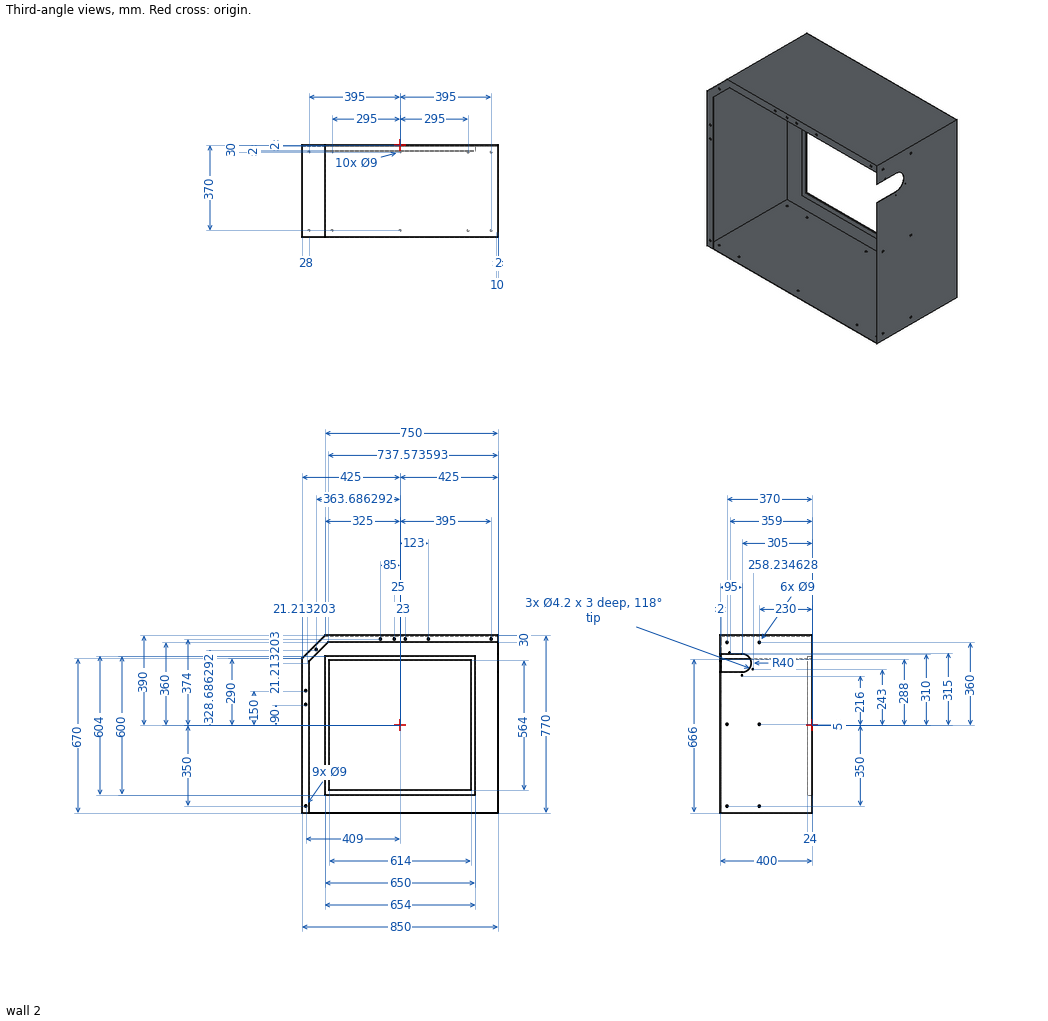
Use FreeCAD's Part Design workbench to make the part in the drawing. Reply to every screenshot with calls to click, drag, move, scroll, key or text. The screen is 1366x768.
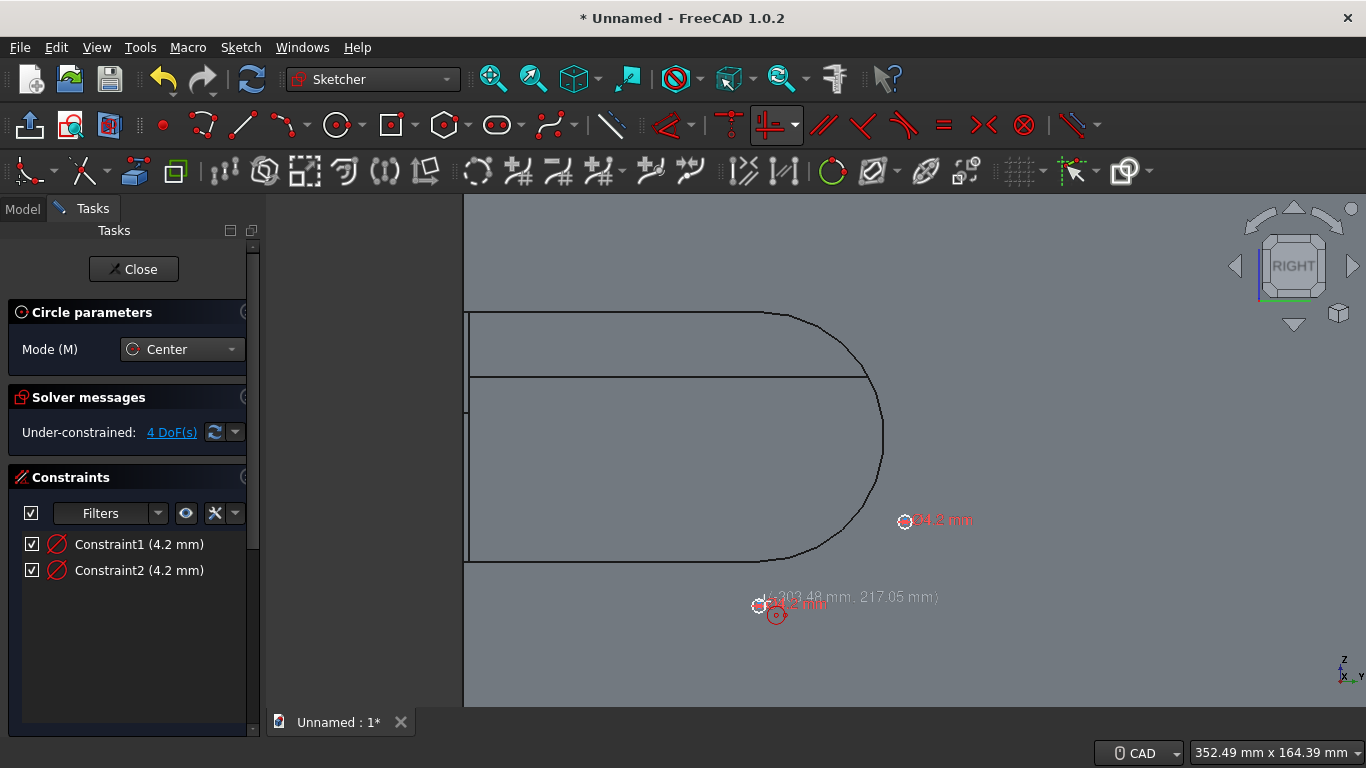
scroll(591, 296, up, 7)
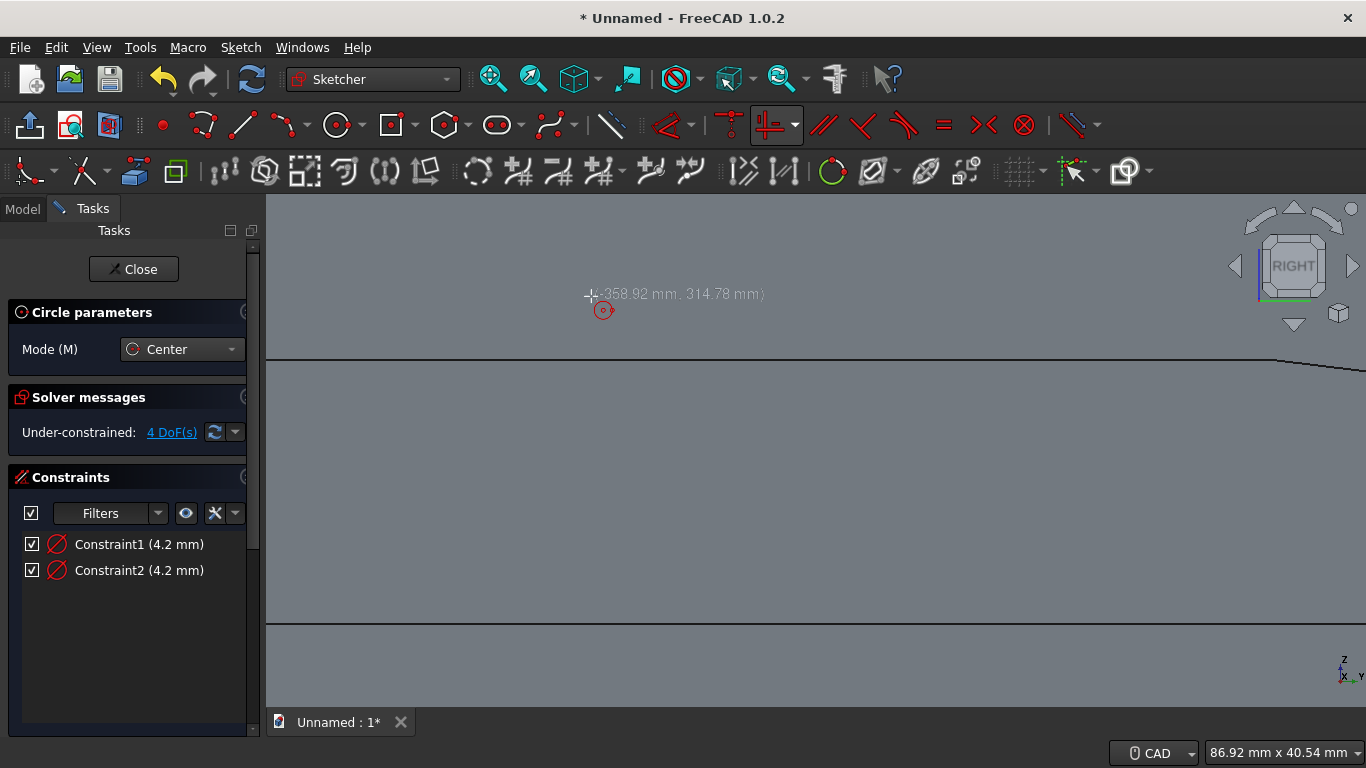
scroll(591, 296, down, 7)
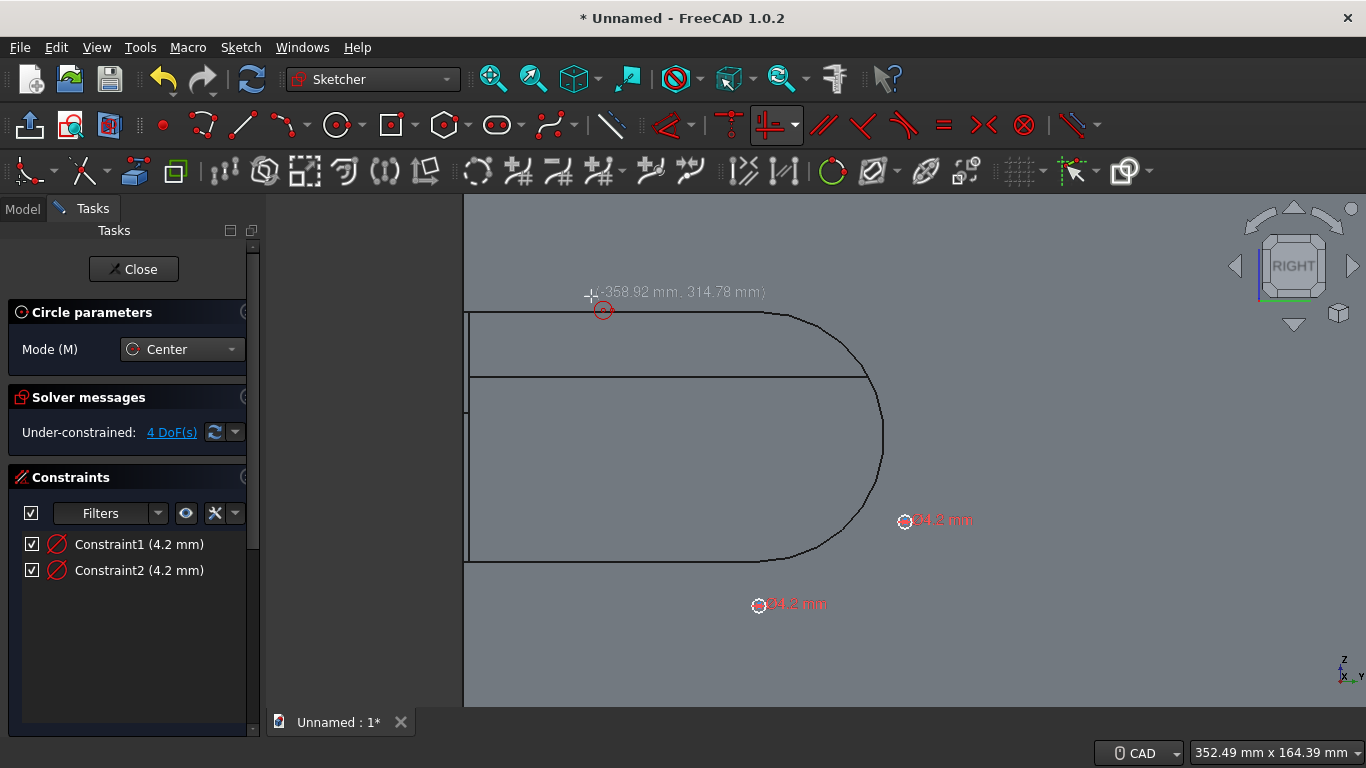
click(591, 296)
move(595, 292)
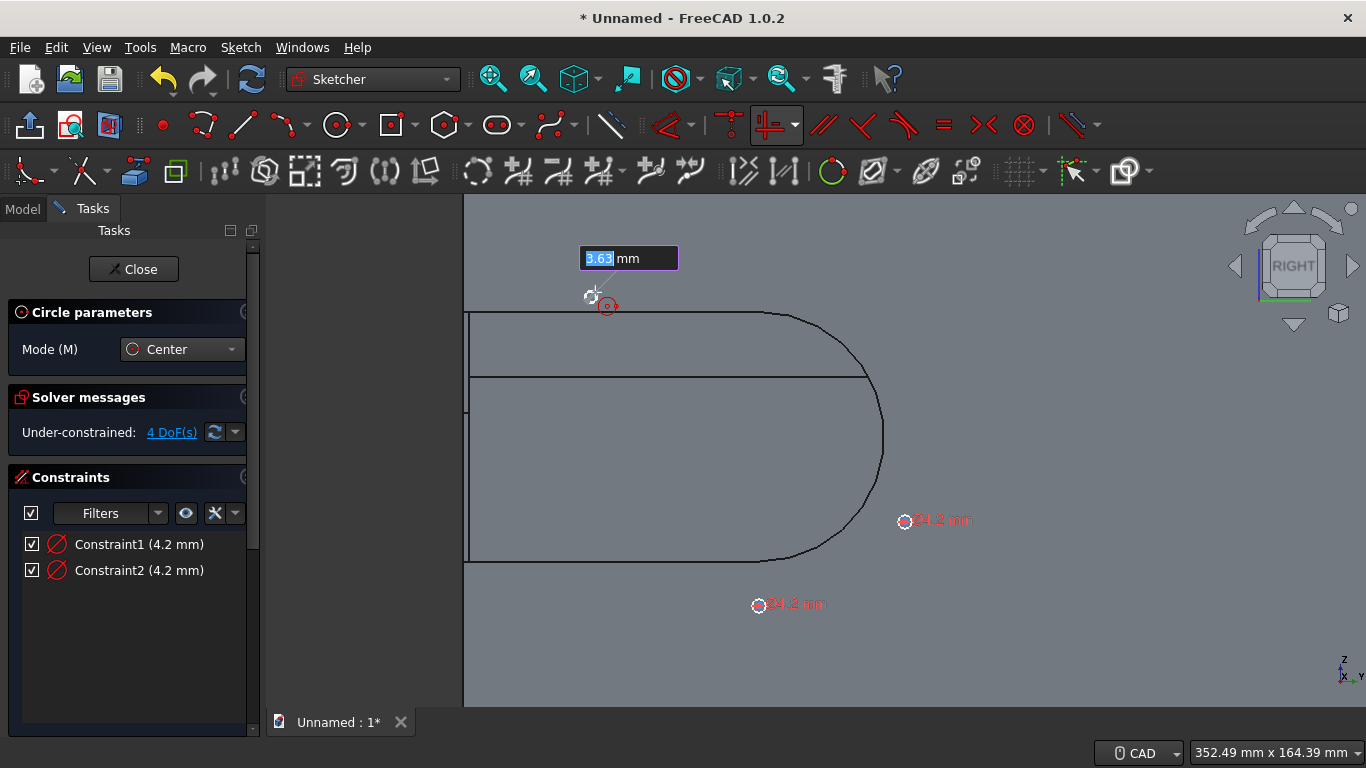
text(4.2)
key(Return)
key(Escape)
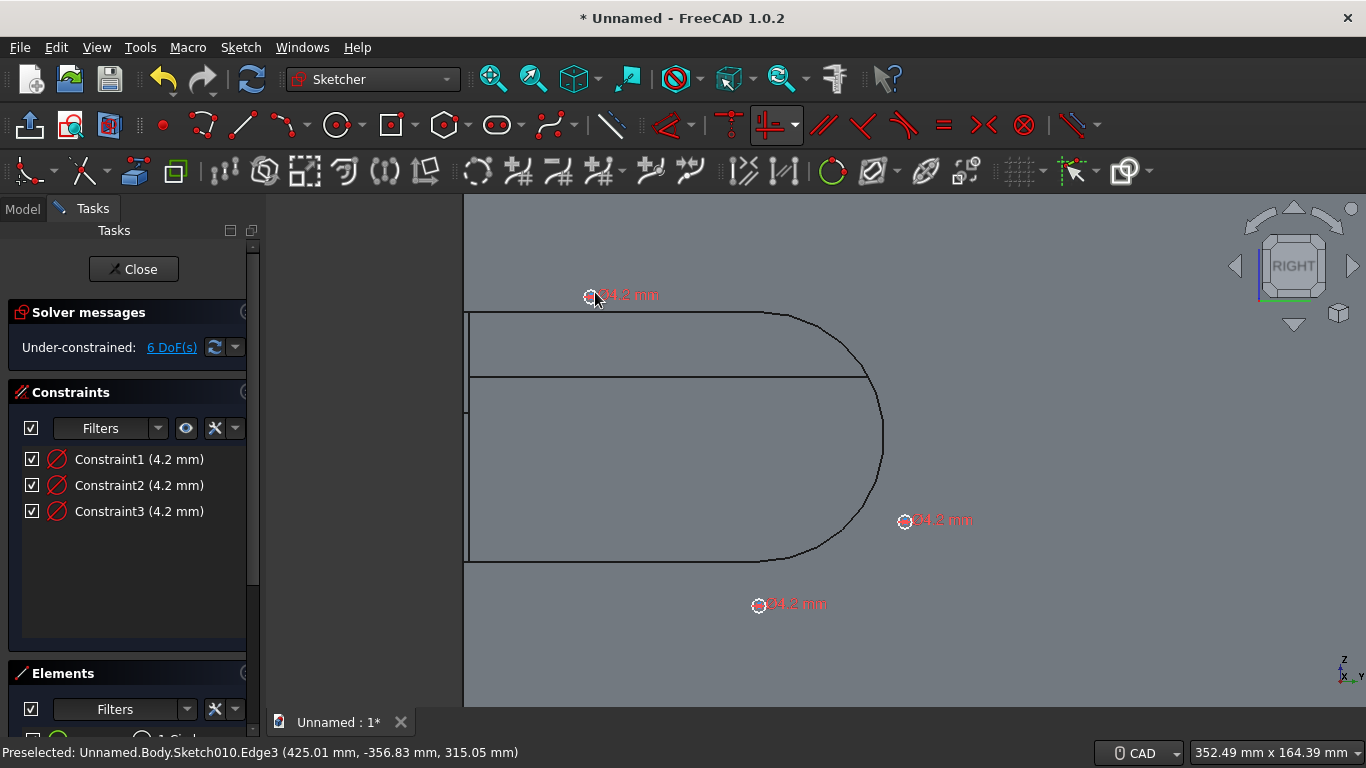
click(666, 126)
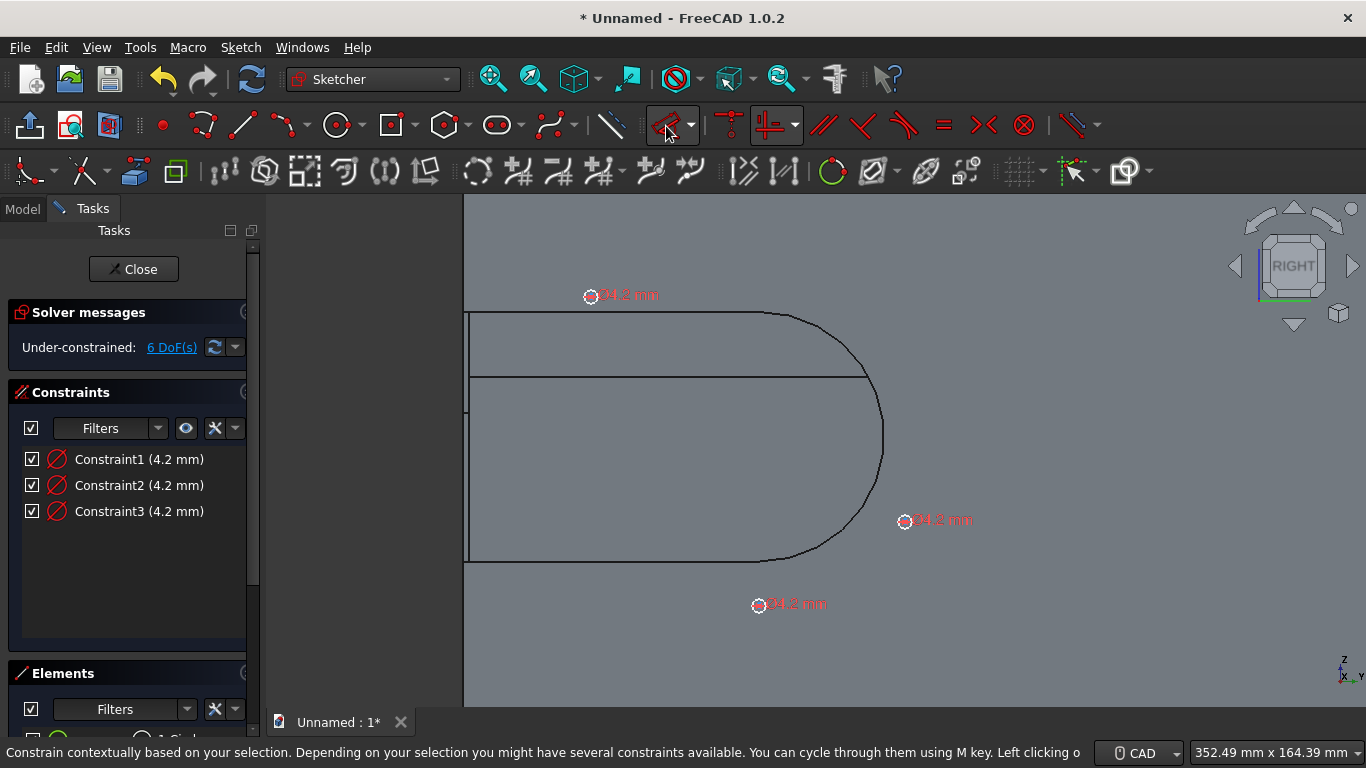
click(905, 522)
click(871, 600)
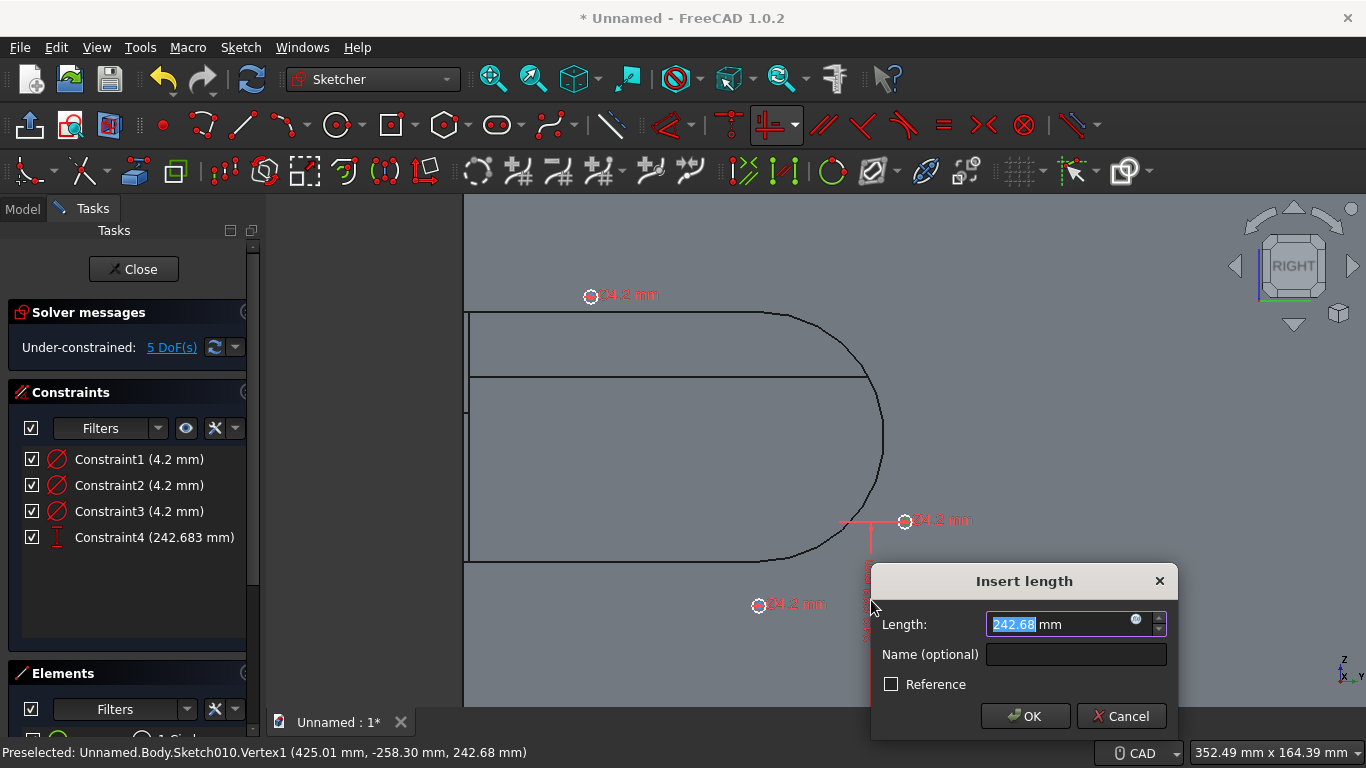
text(243)
key(Return)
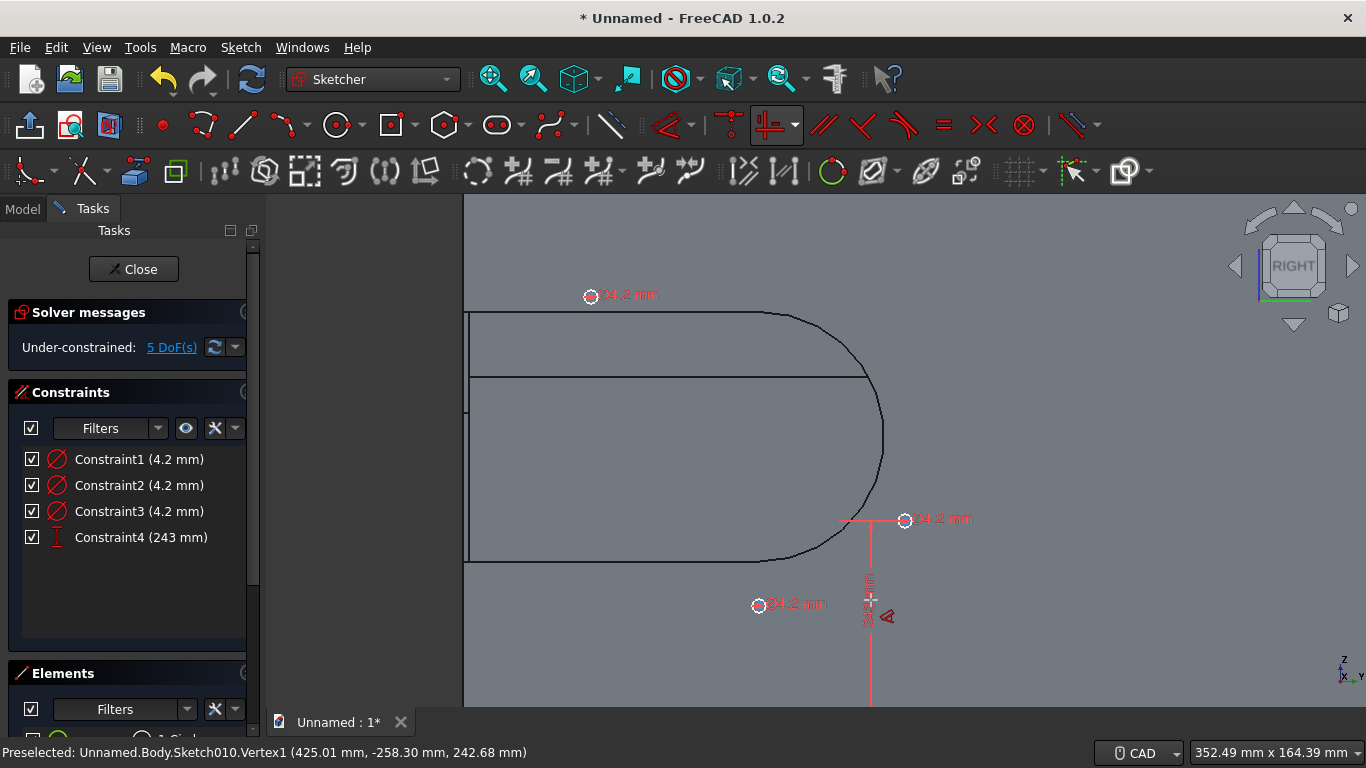
click(759, 606)
click(980, 572)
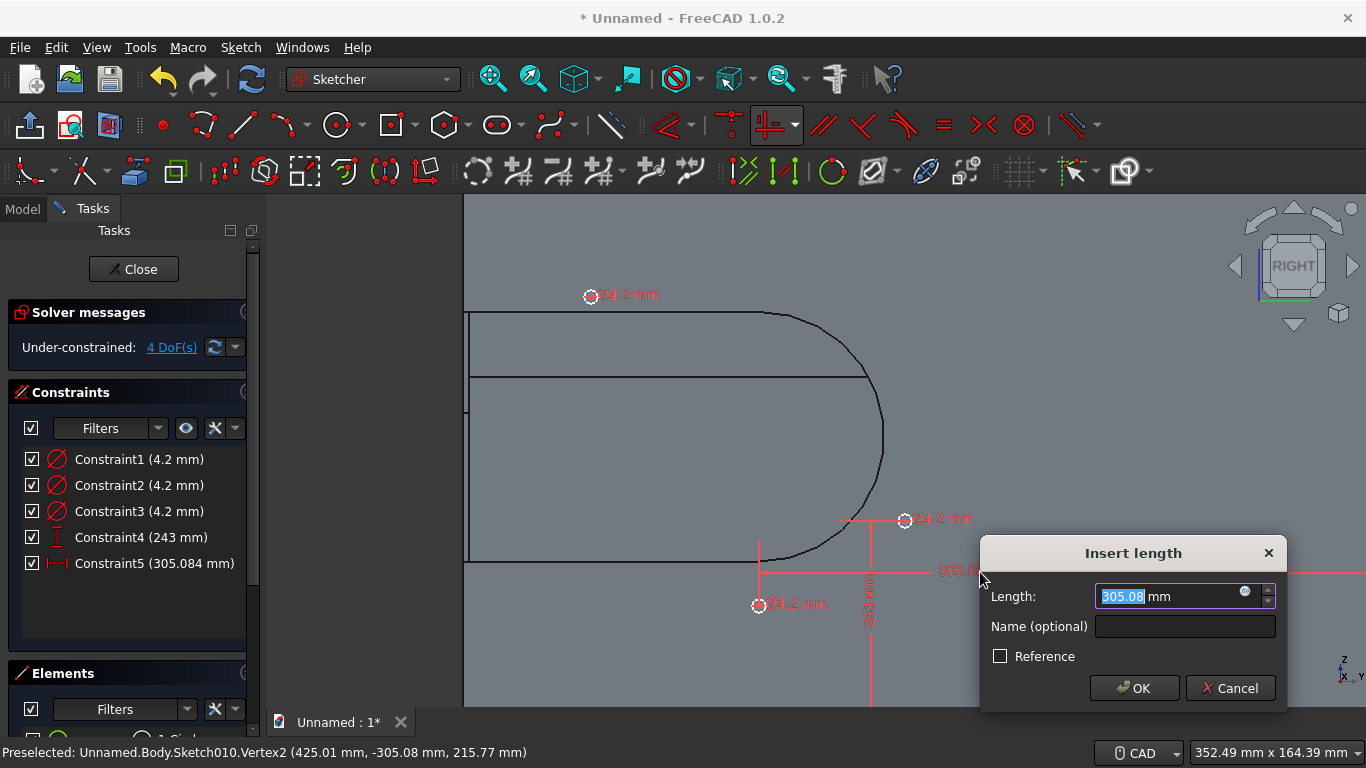
text(305)
key(Return)